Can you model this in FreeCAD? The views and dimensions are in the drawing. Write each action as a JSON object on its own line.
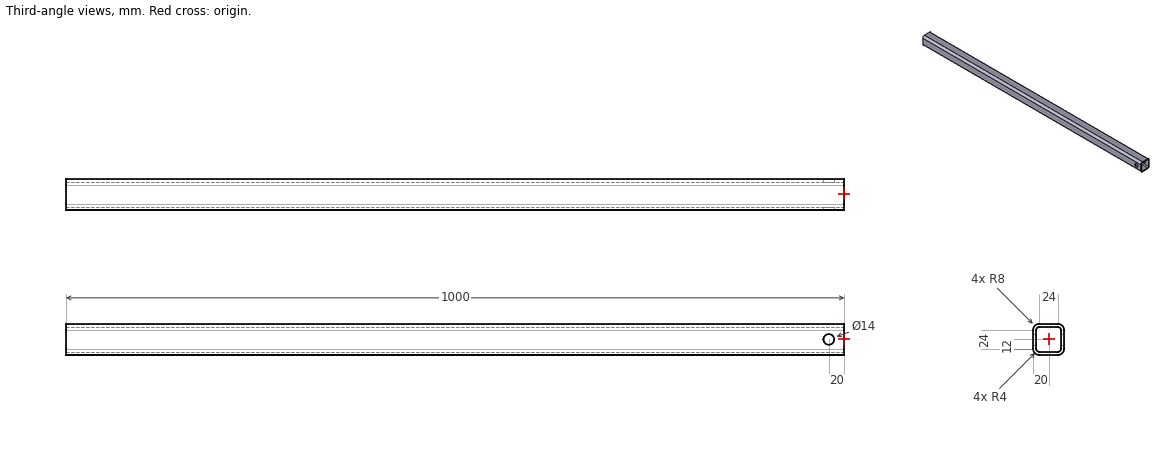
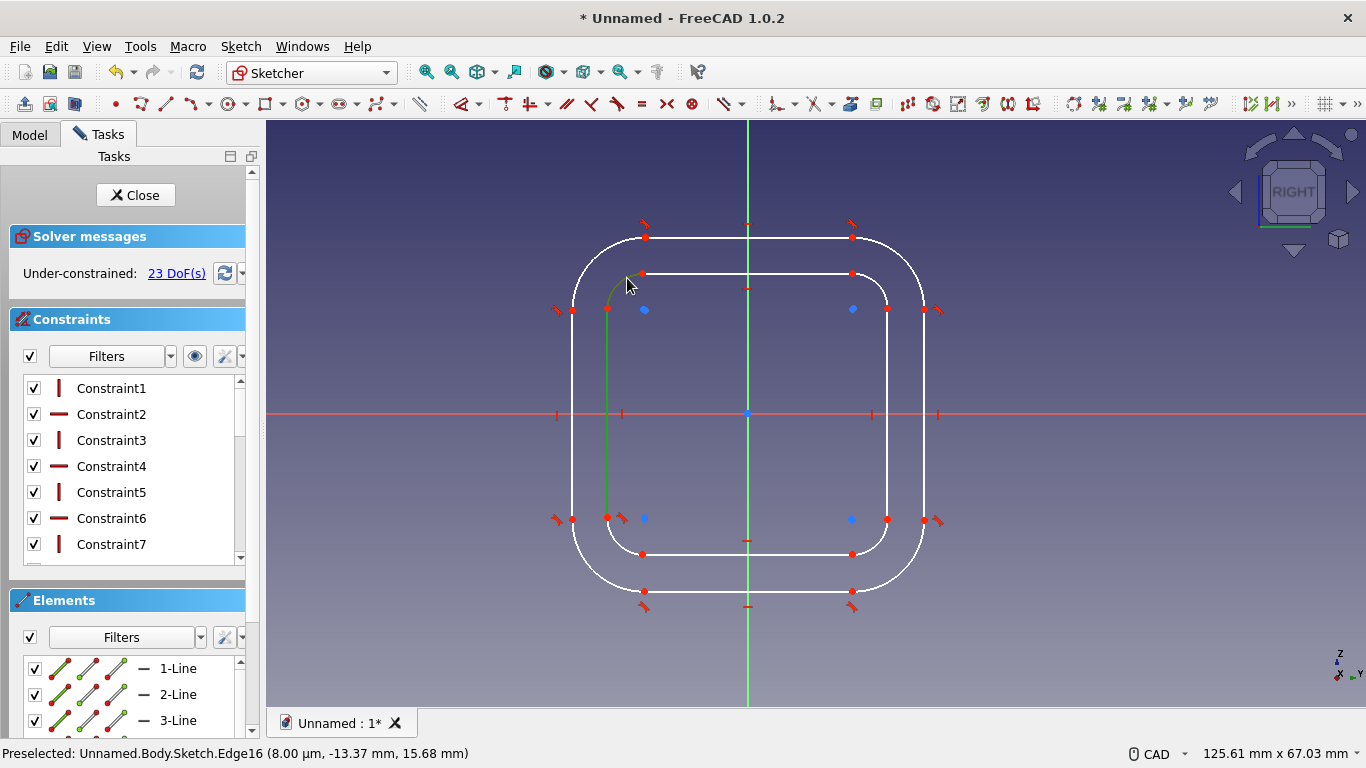
{"action": "left_click", "coordinate": [617, 104]}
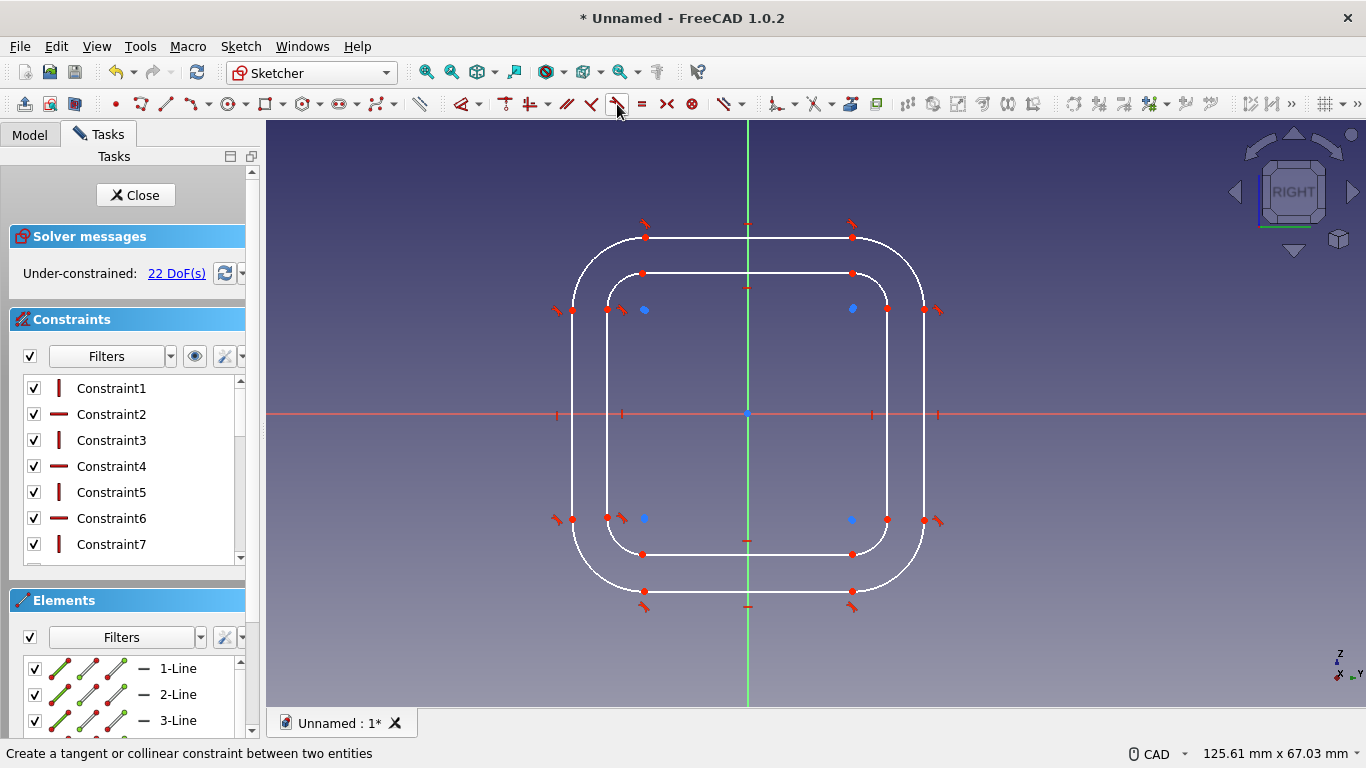
{"action": "left_click", "coordinate": [705, 555]}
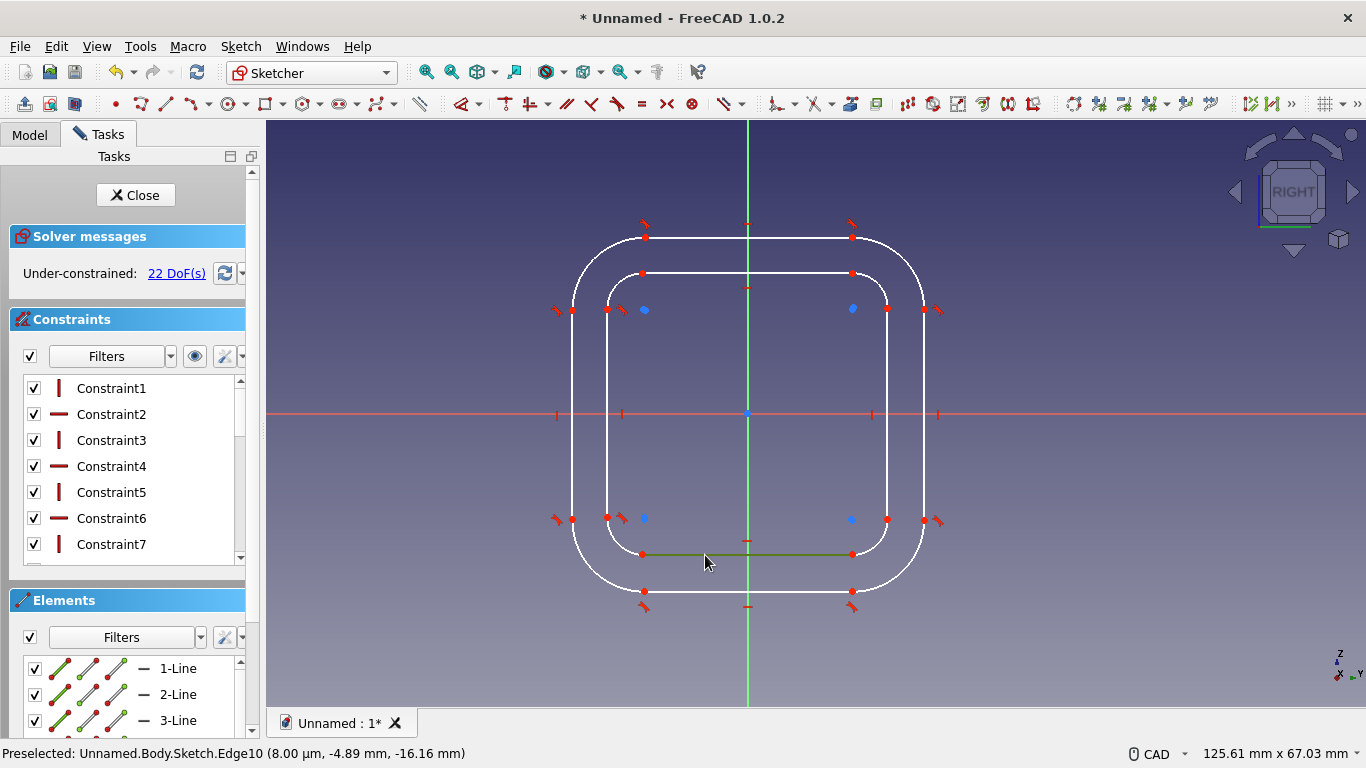
{"action": "left_click", "coordinate": [611, 534]}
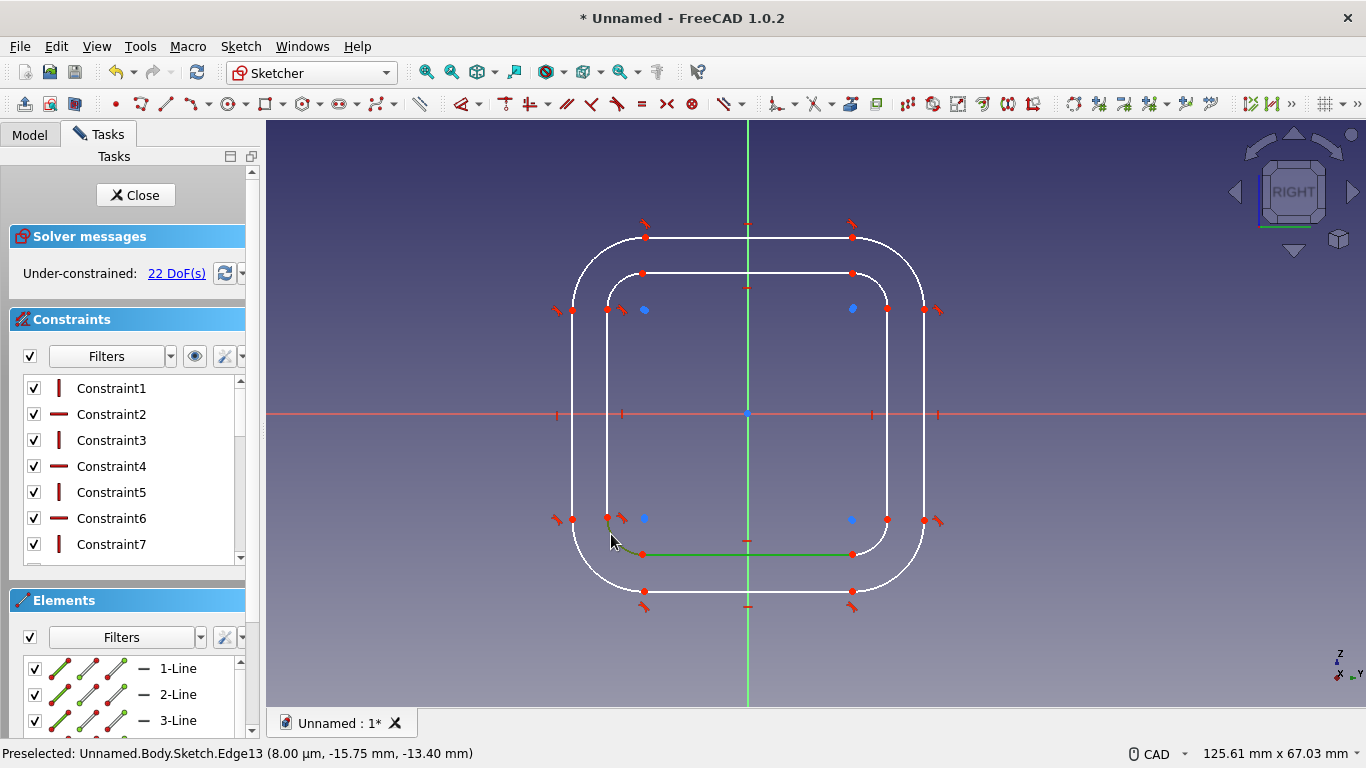
{"action": "left_click", "coordinate": [617, 104]}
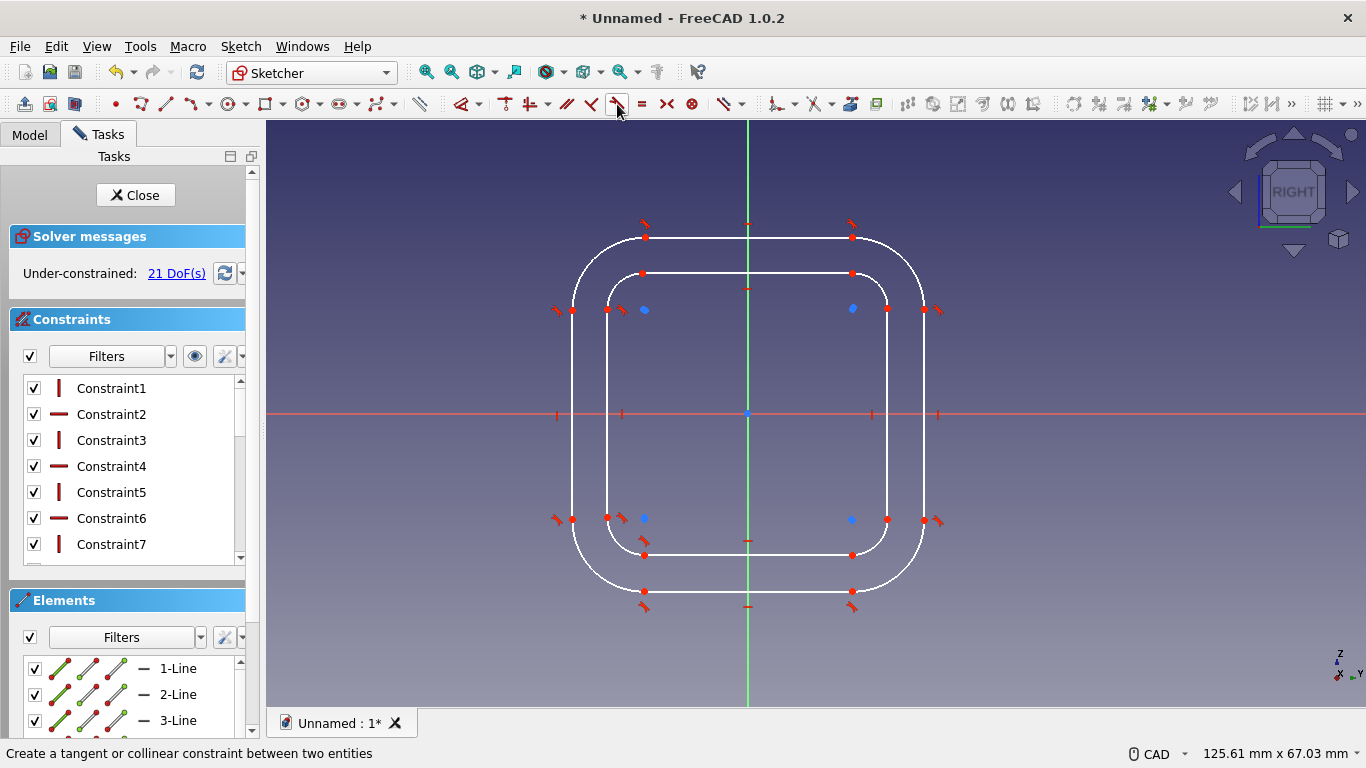
{"action": "left_click", "coordinate": [707, 555]}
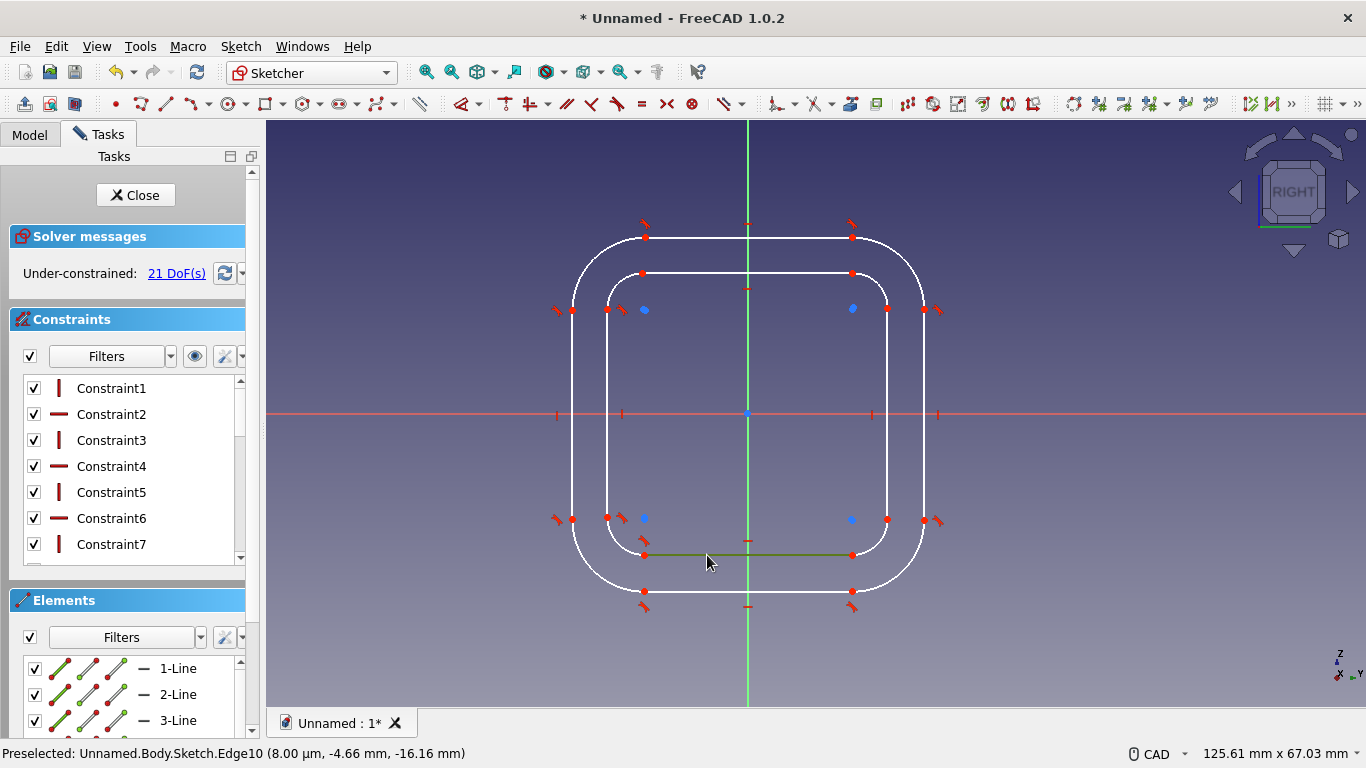
{"action": "left_click", "coordinate": [868, 551]}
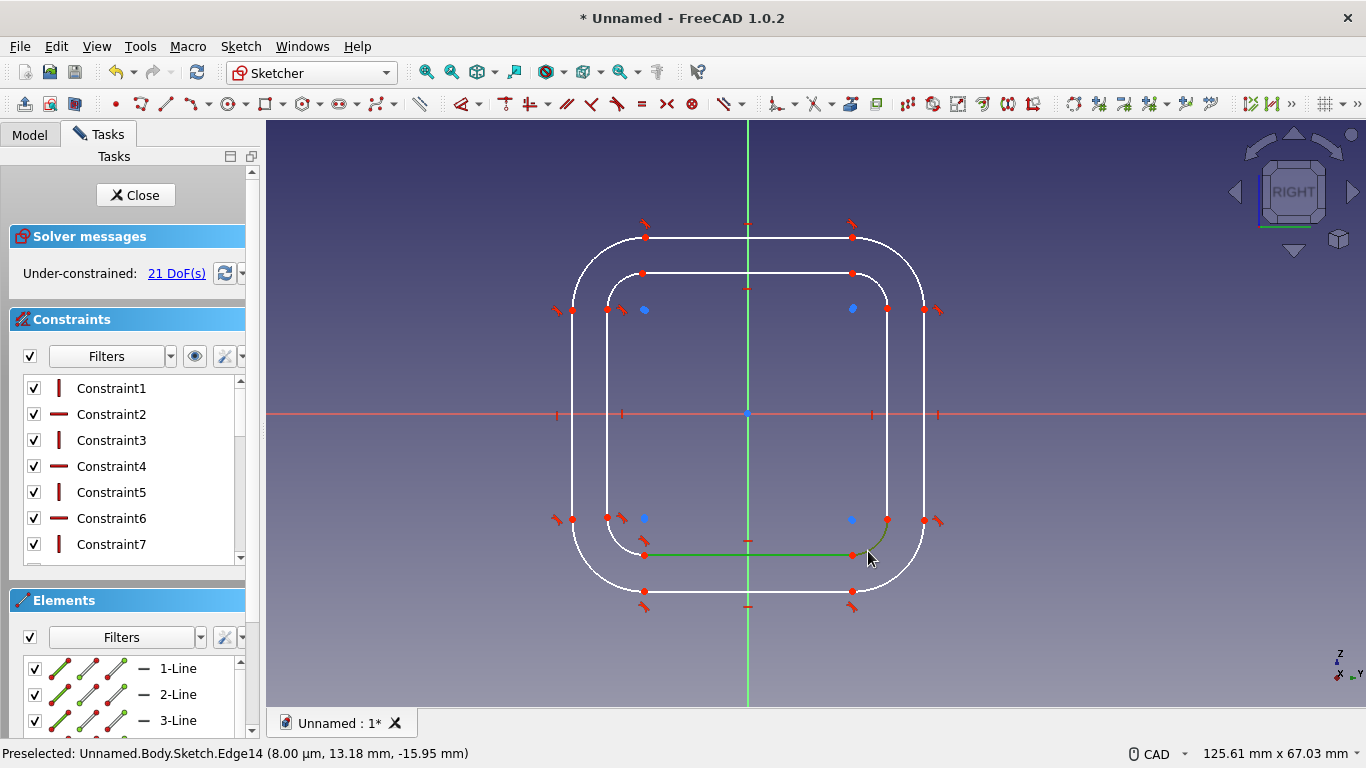
{"action": "left_click", "coordinate": [617, 104]}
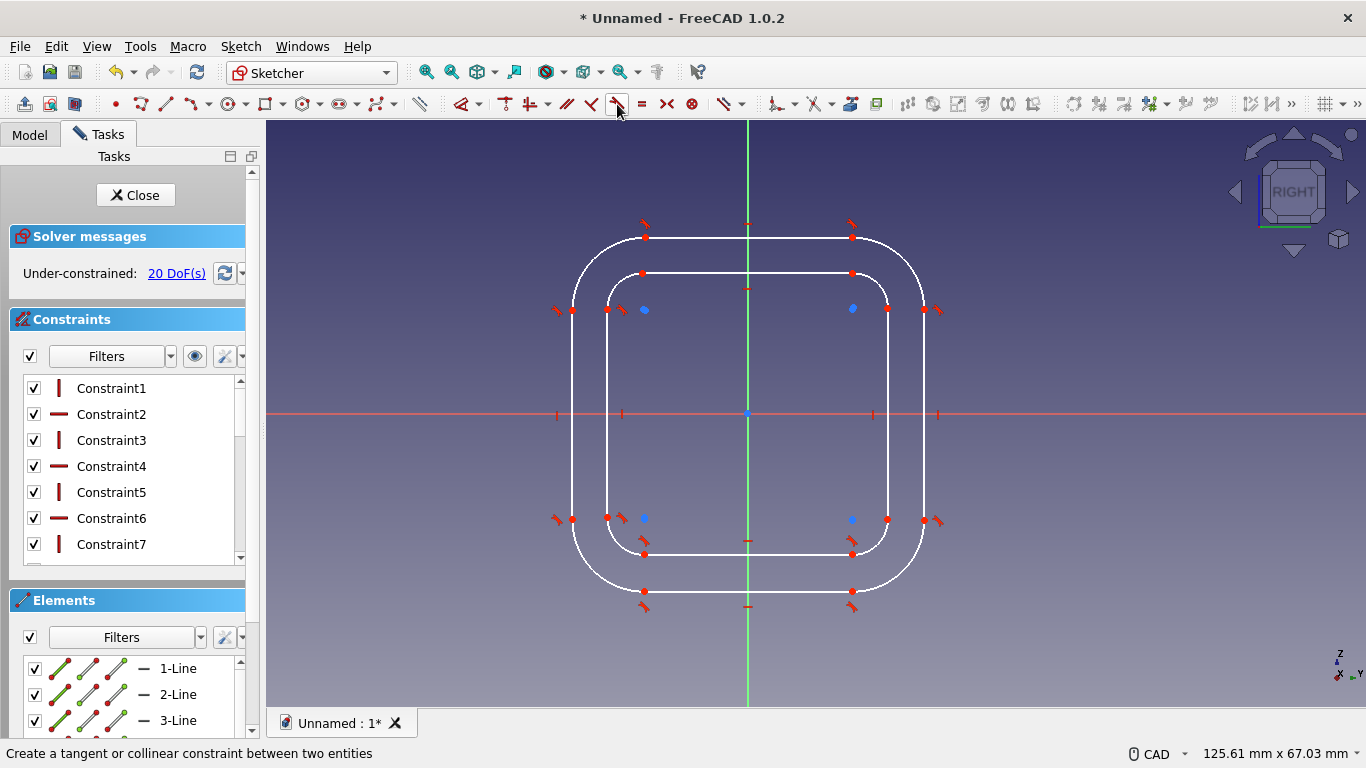
{"action": "left_click", "coordinate": [888, 457]}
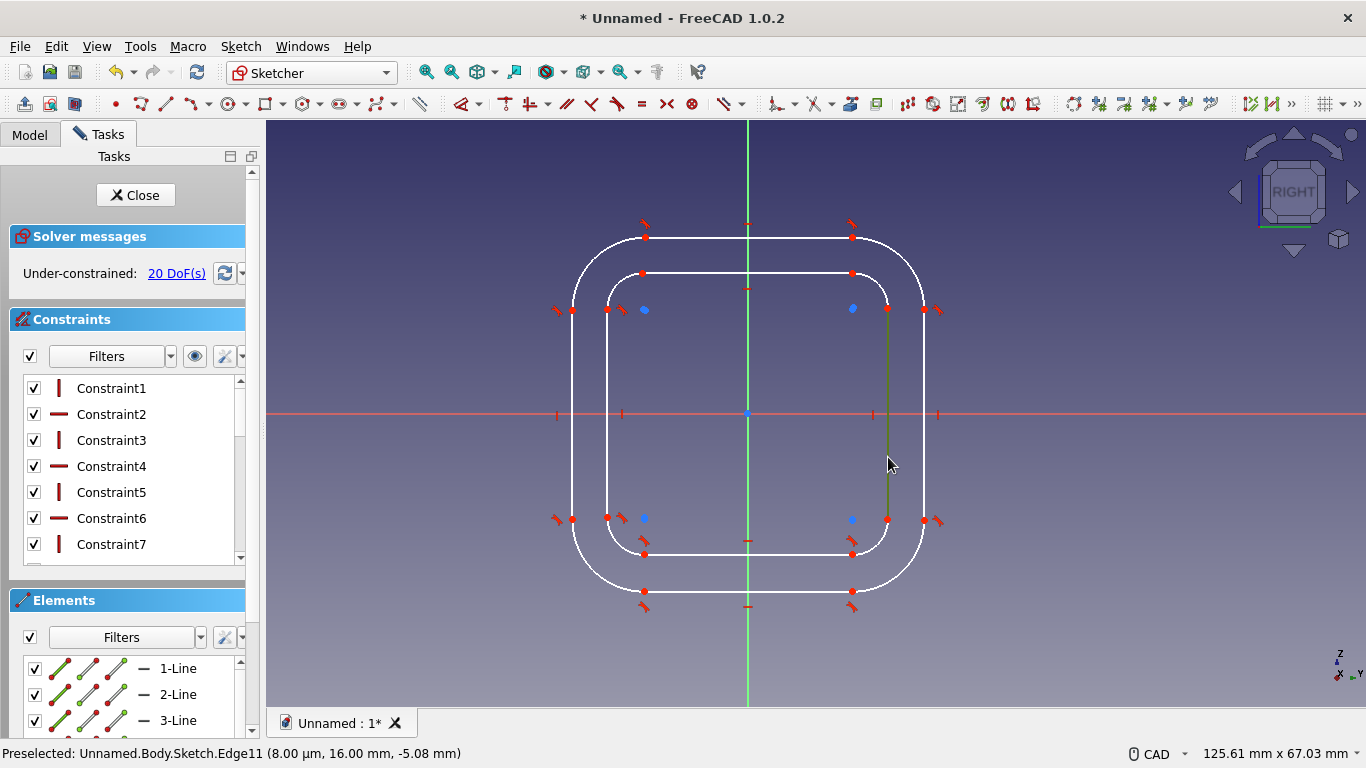
{"action": "left_click", "coordinate": [868, 551]}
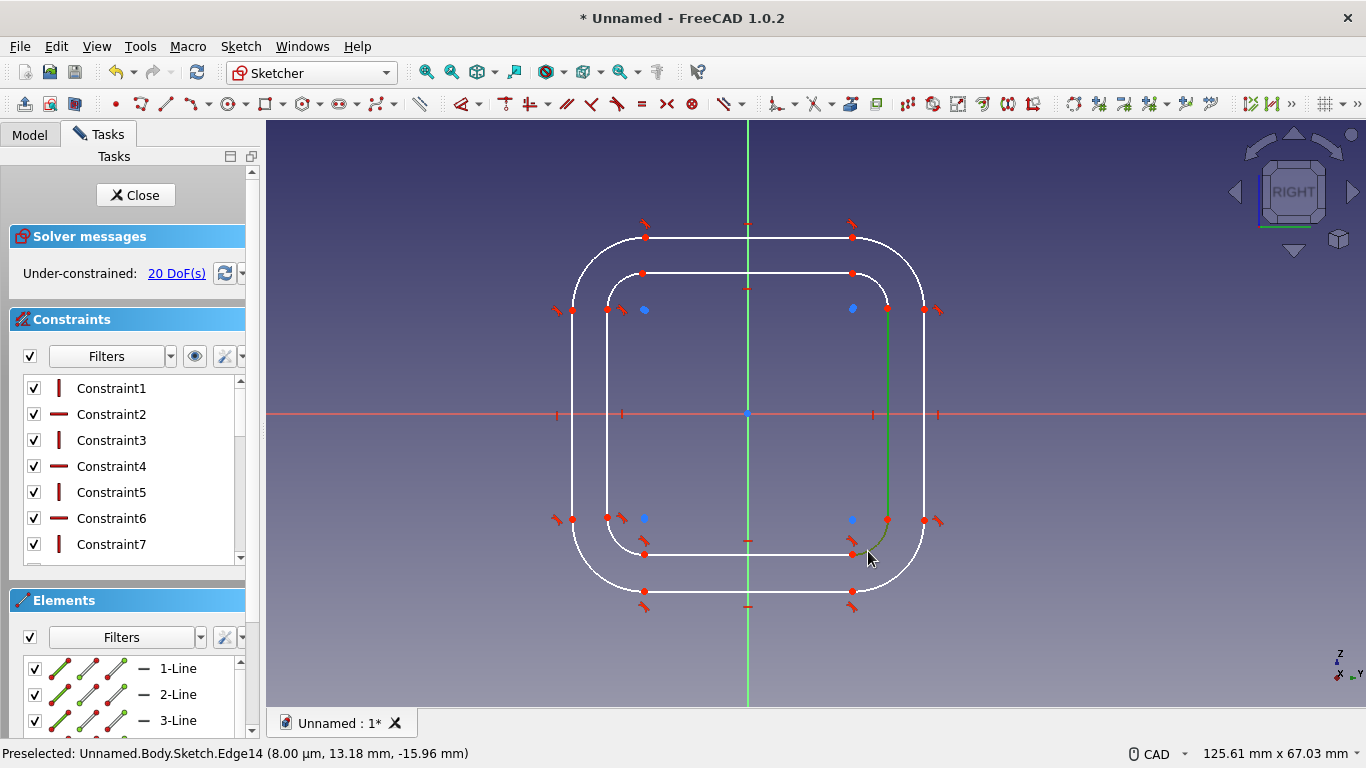
{"action": "left_click", "coordinate": [617, 104]}